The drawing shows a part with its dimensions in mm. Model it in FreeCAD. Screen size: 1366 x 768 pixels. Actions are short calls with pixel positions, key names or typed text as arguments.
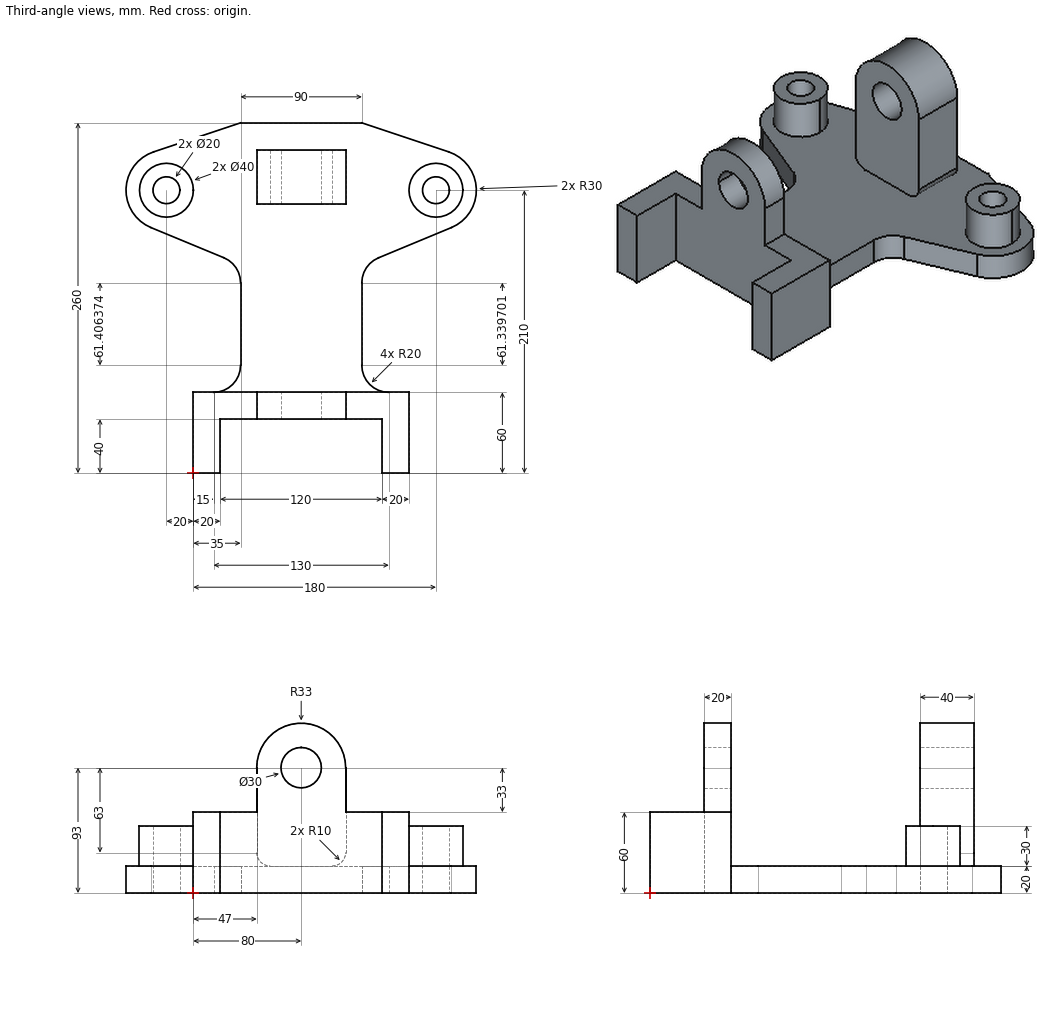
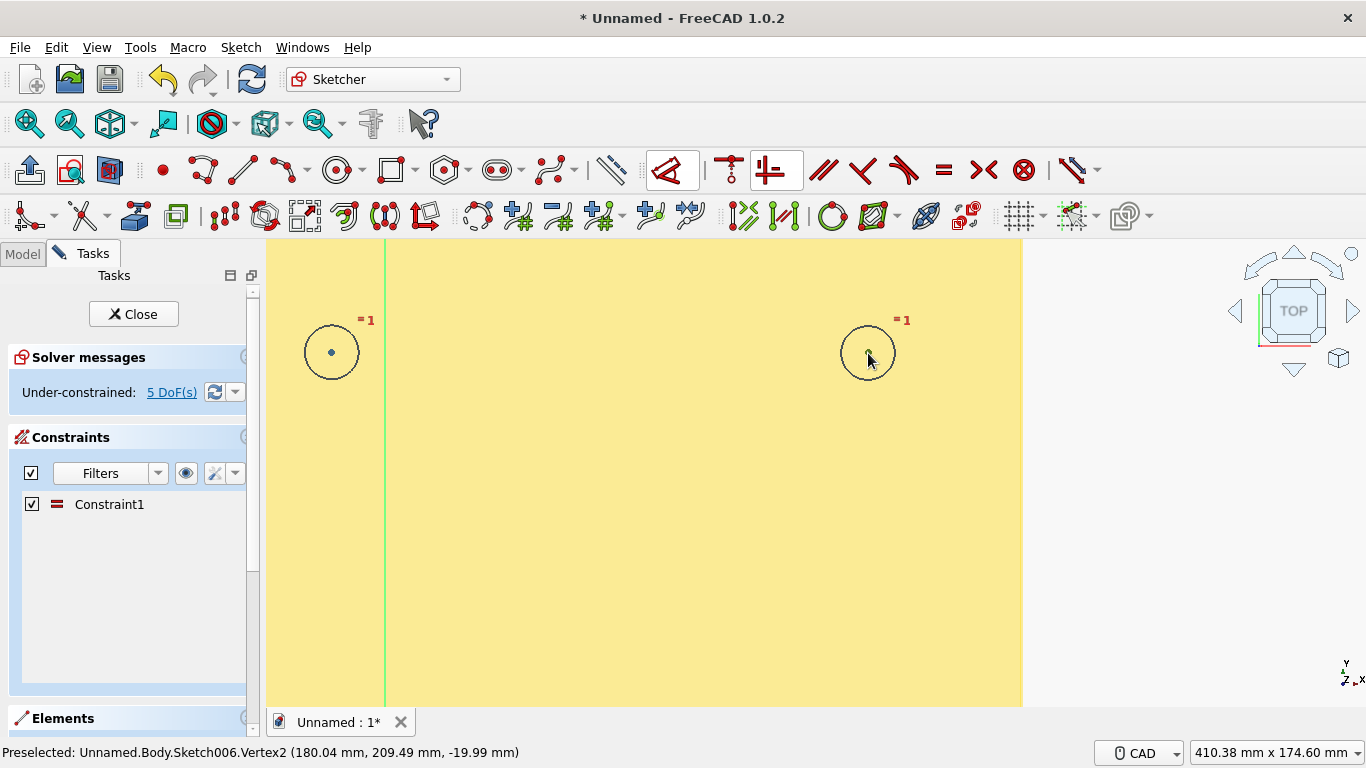
key(h)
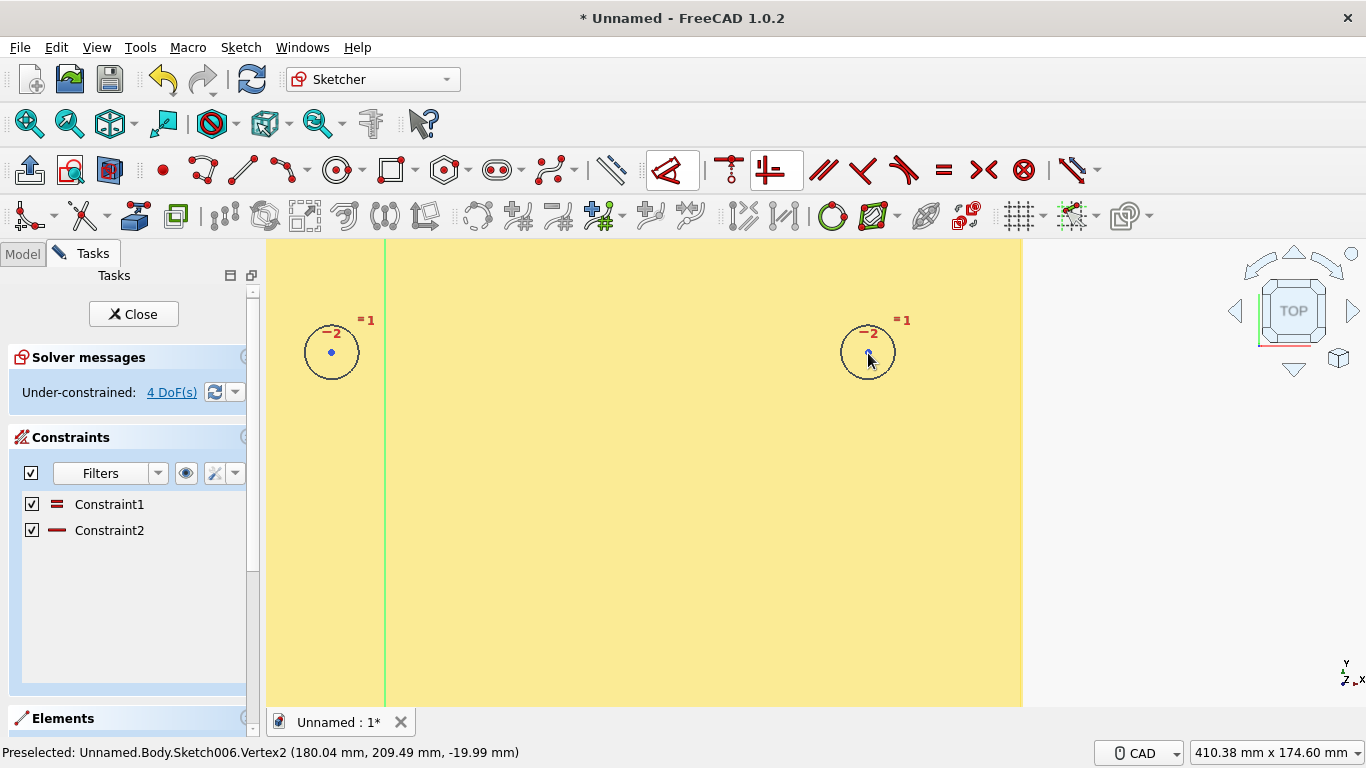
click(351, 333)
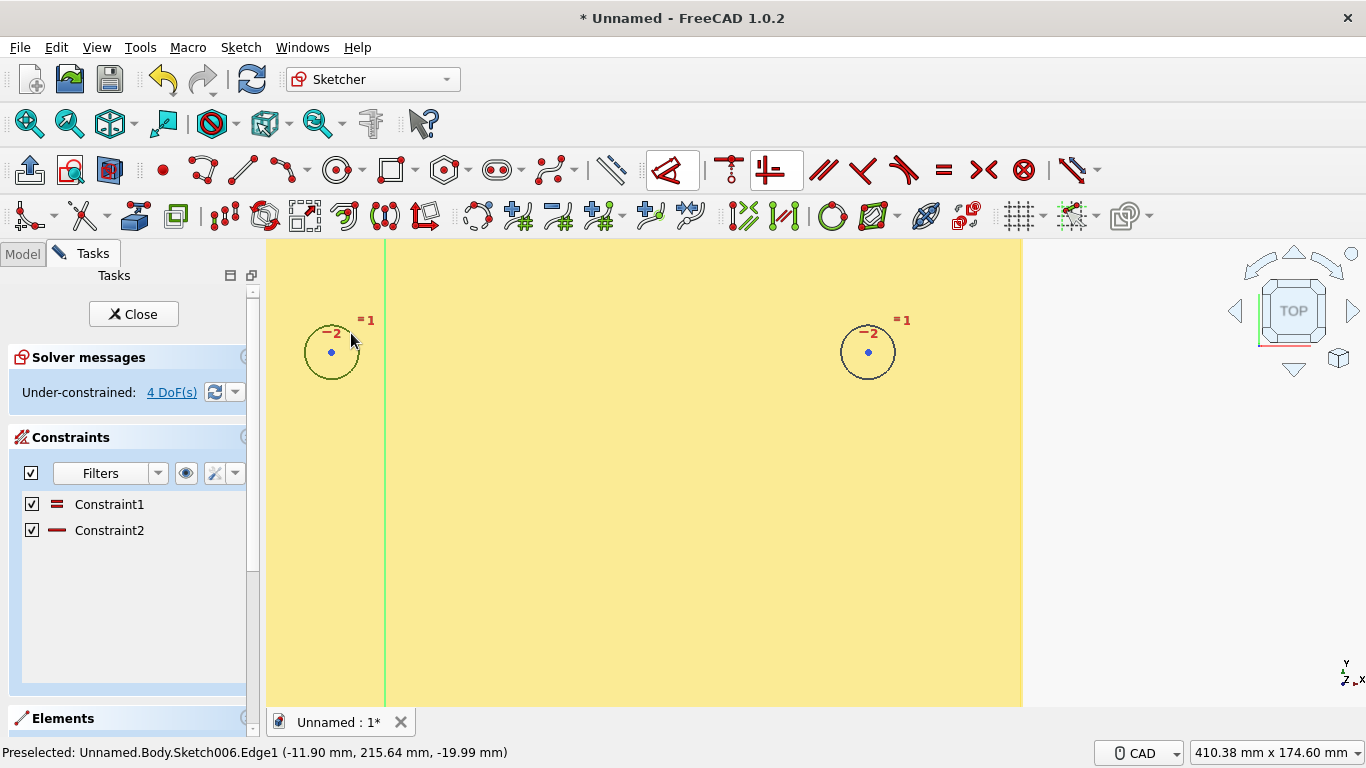
click(694, 170)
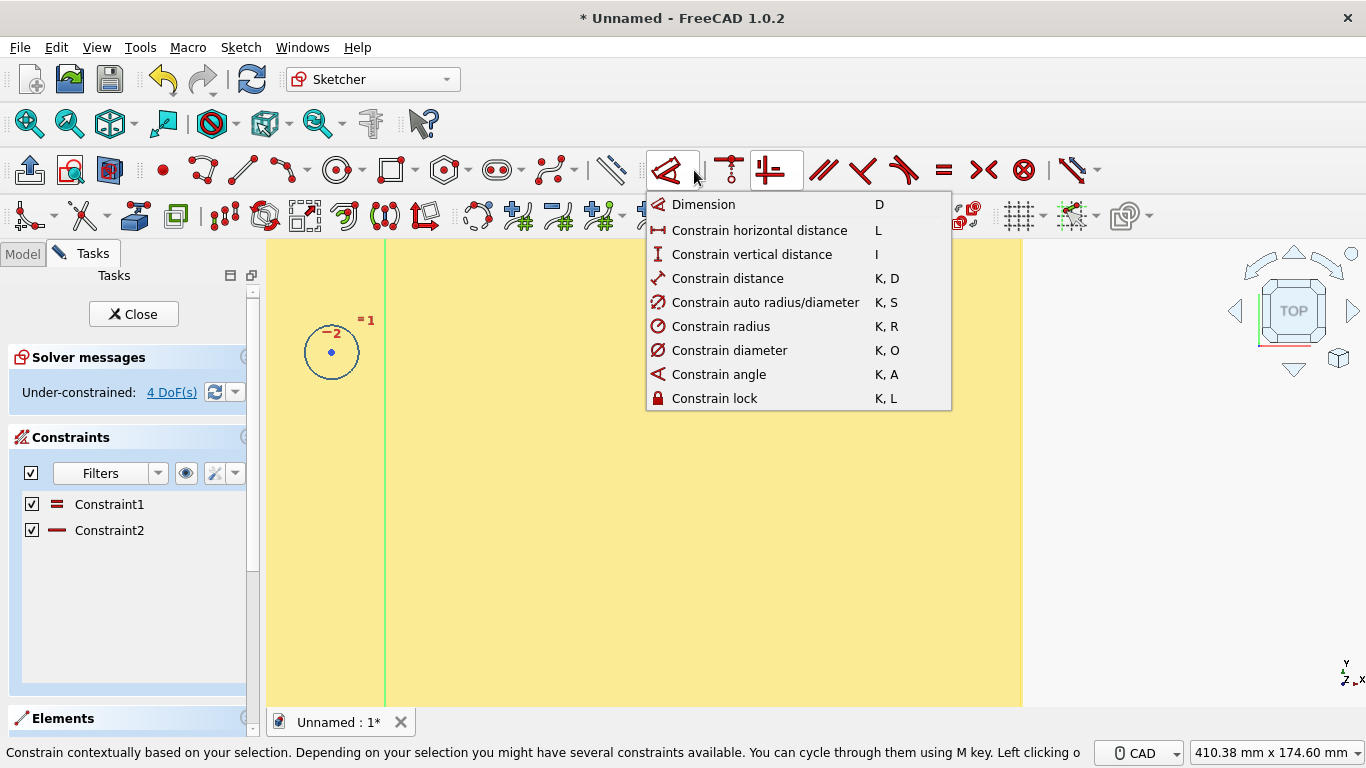
click(799, 350)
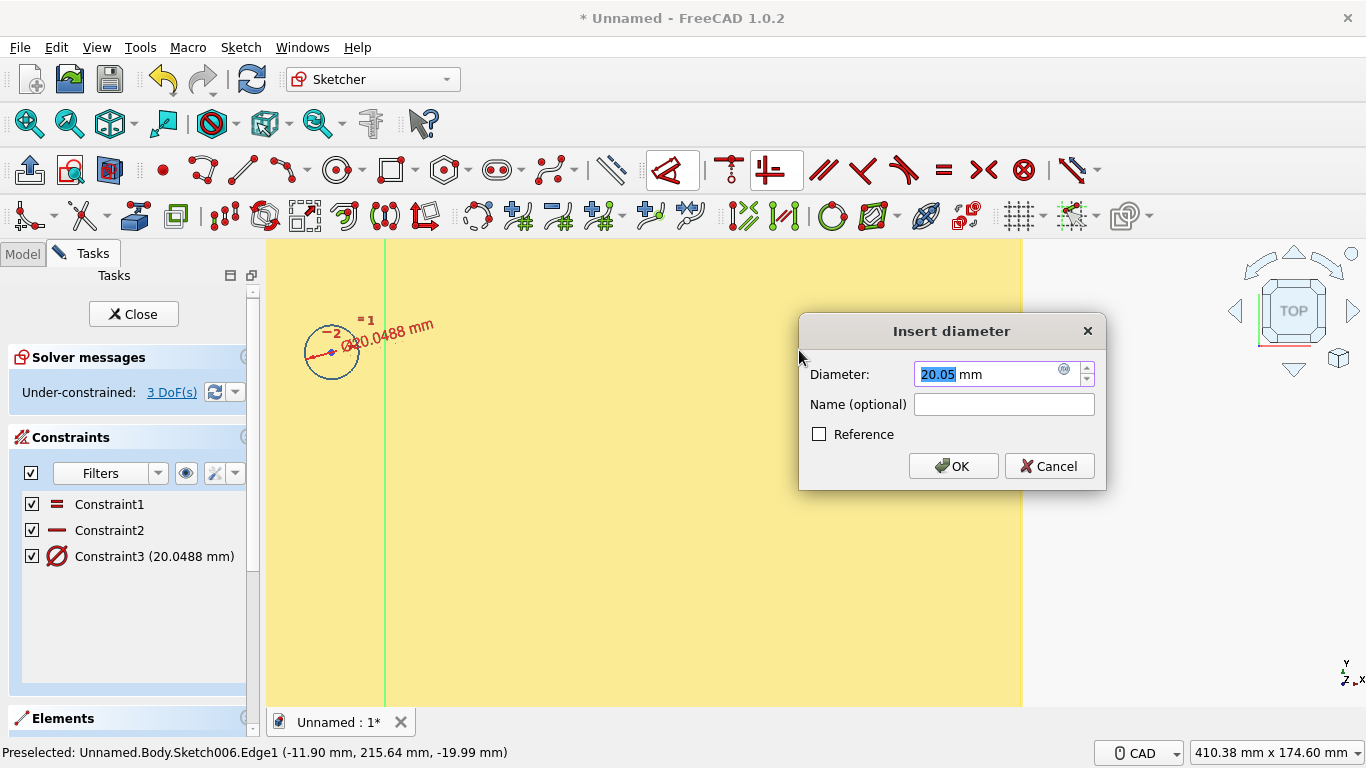
text(20)
key(Return)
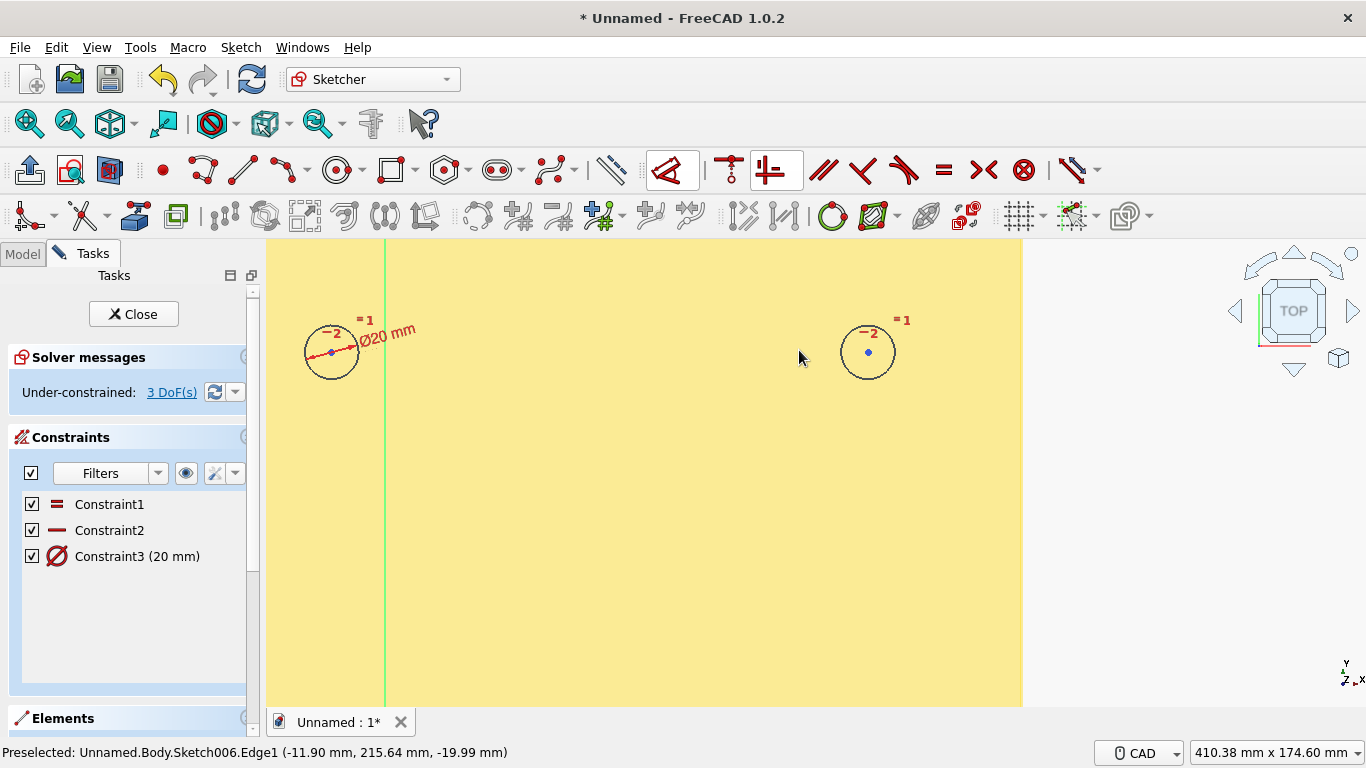
click(332, 352)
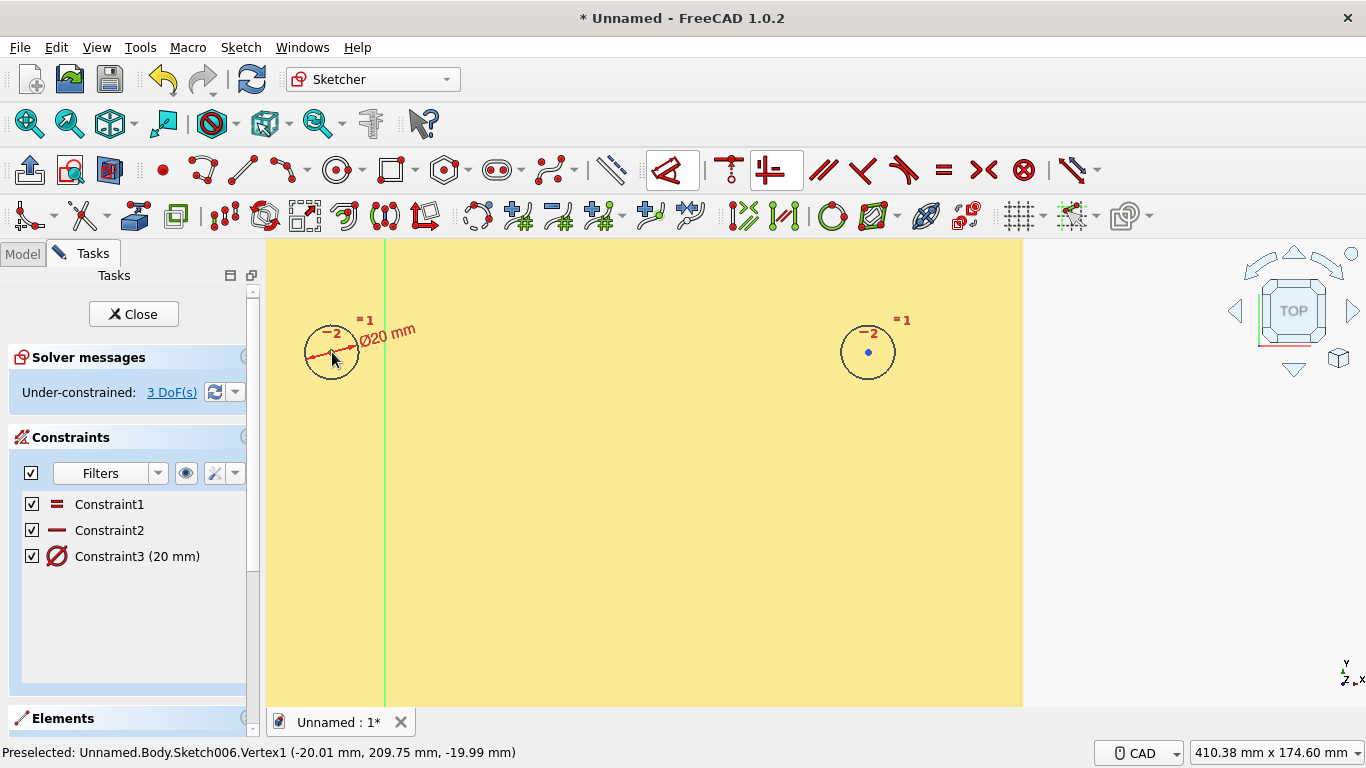
click(694, 170)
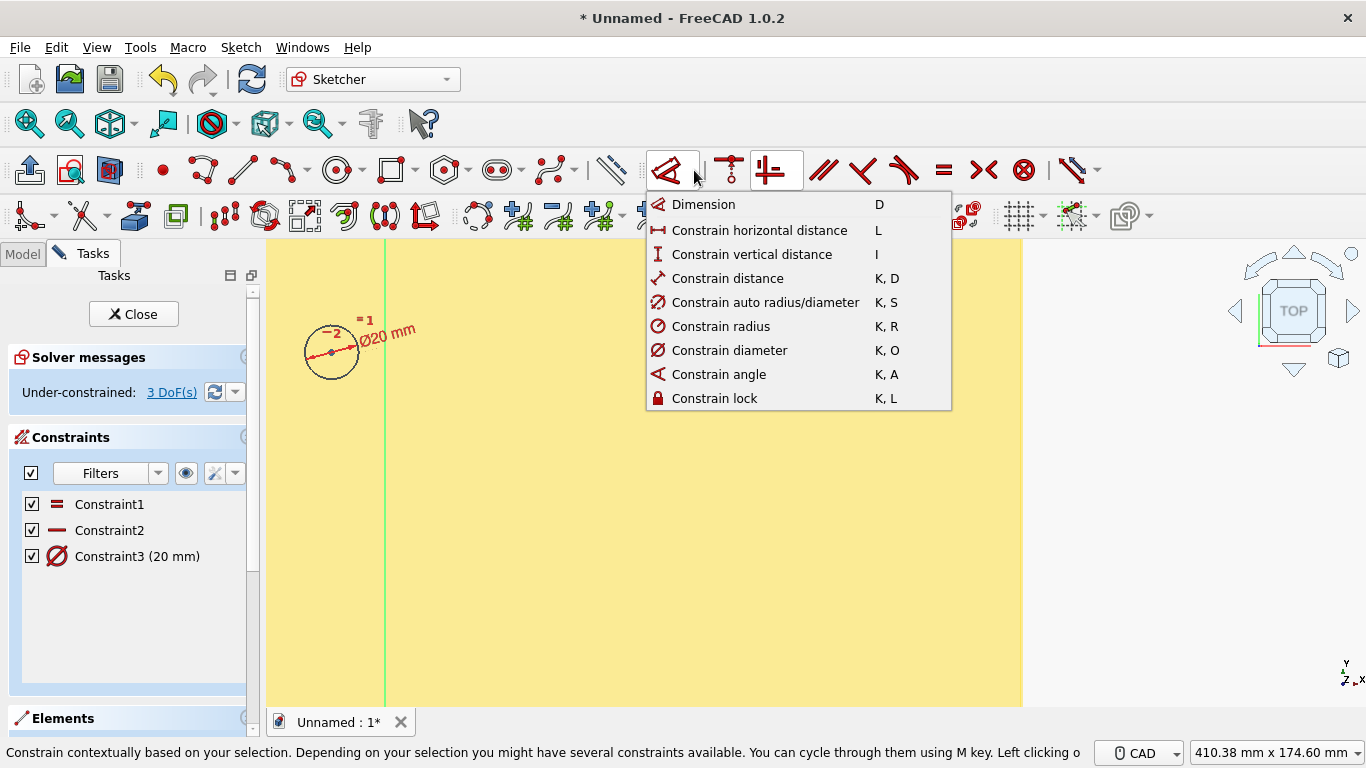
click(799, 230)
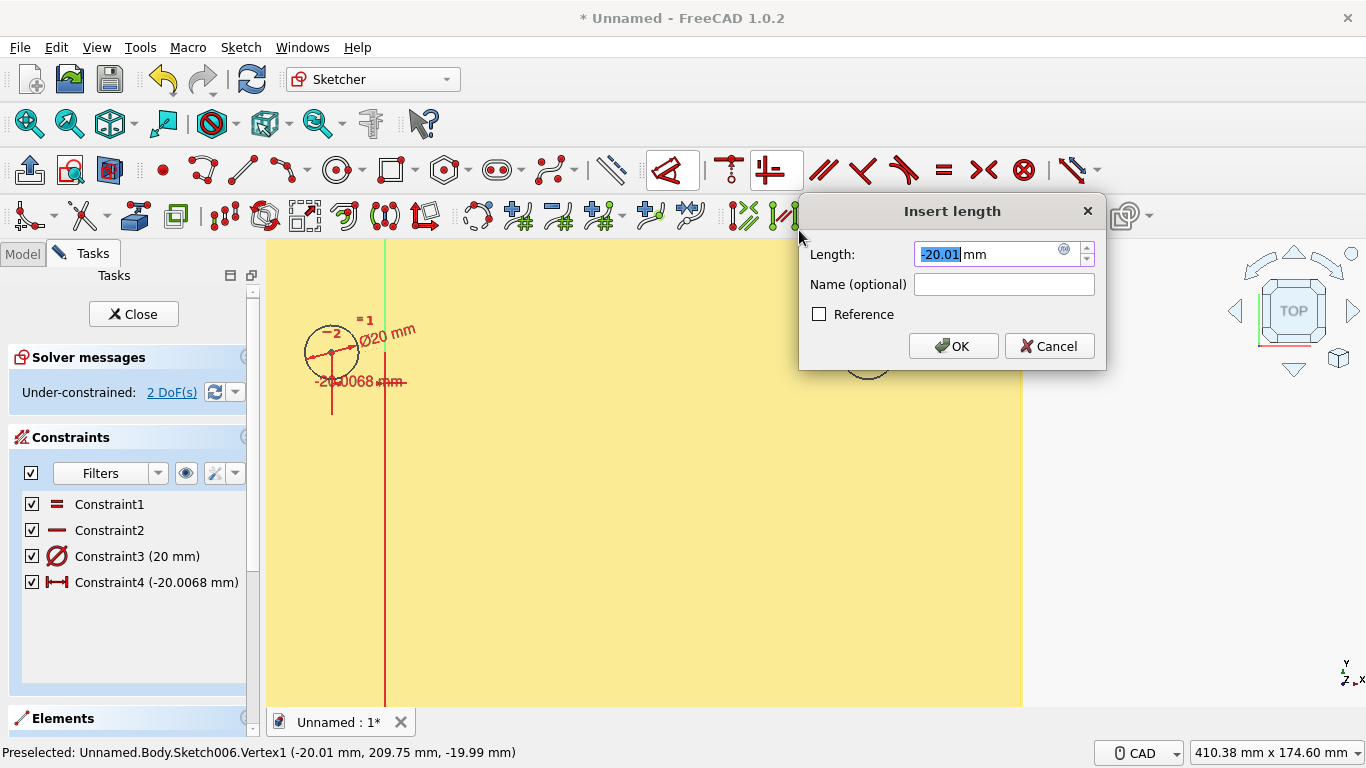
text(-20)
key(Return)